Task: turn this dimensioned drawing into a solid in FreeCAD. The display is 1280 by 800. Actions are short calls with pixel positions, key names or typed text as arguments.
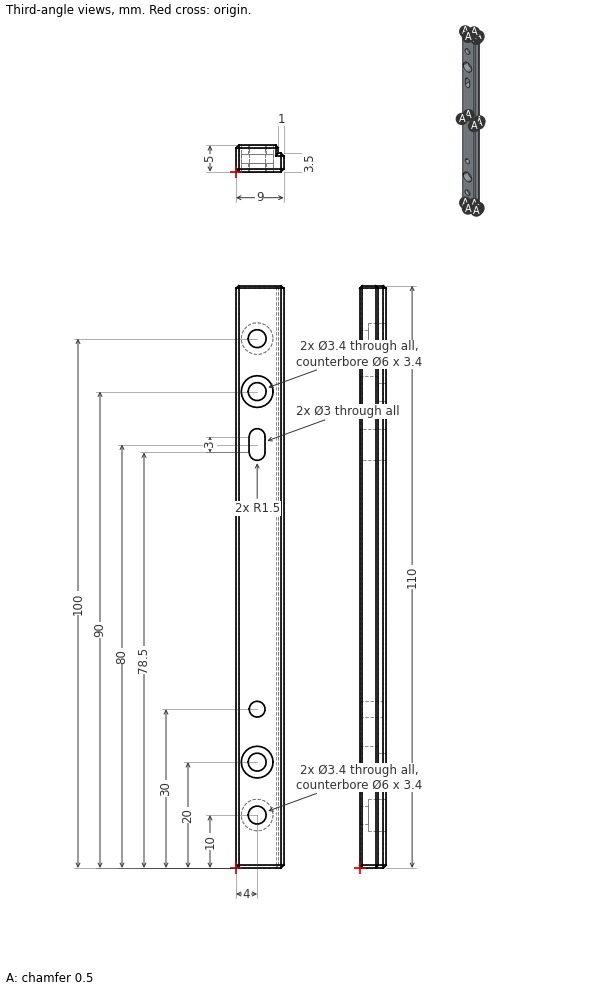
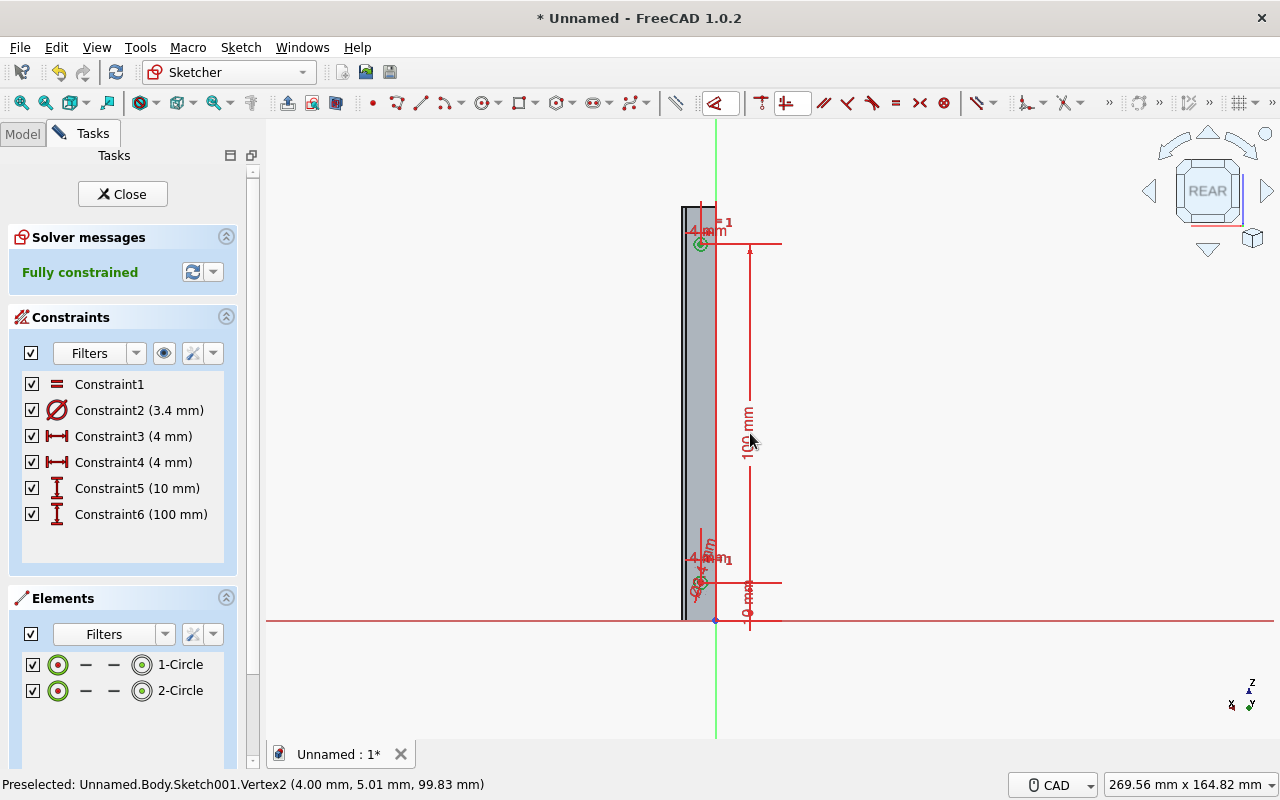
click(123, 194)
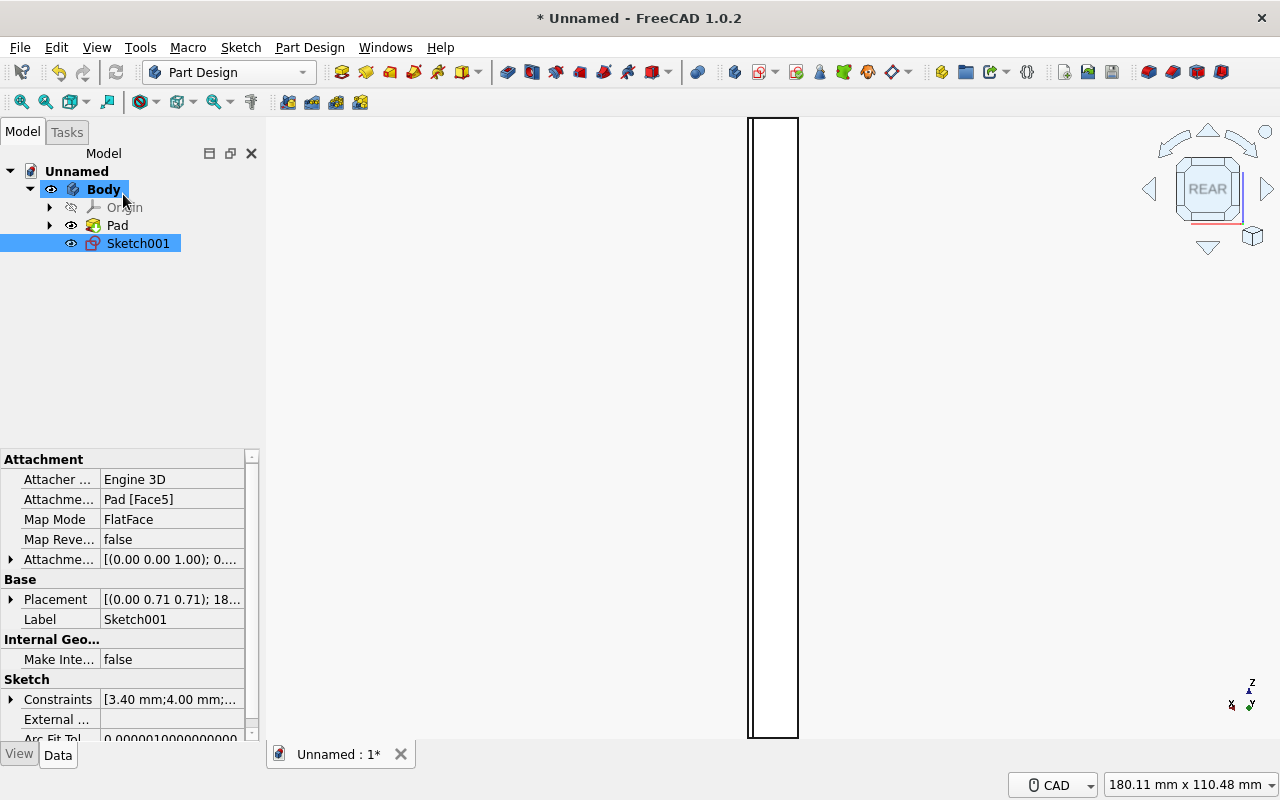
click(532, 72)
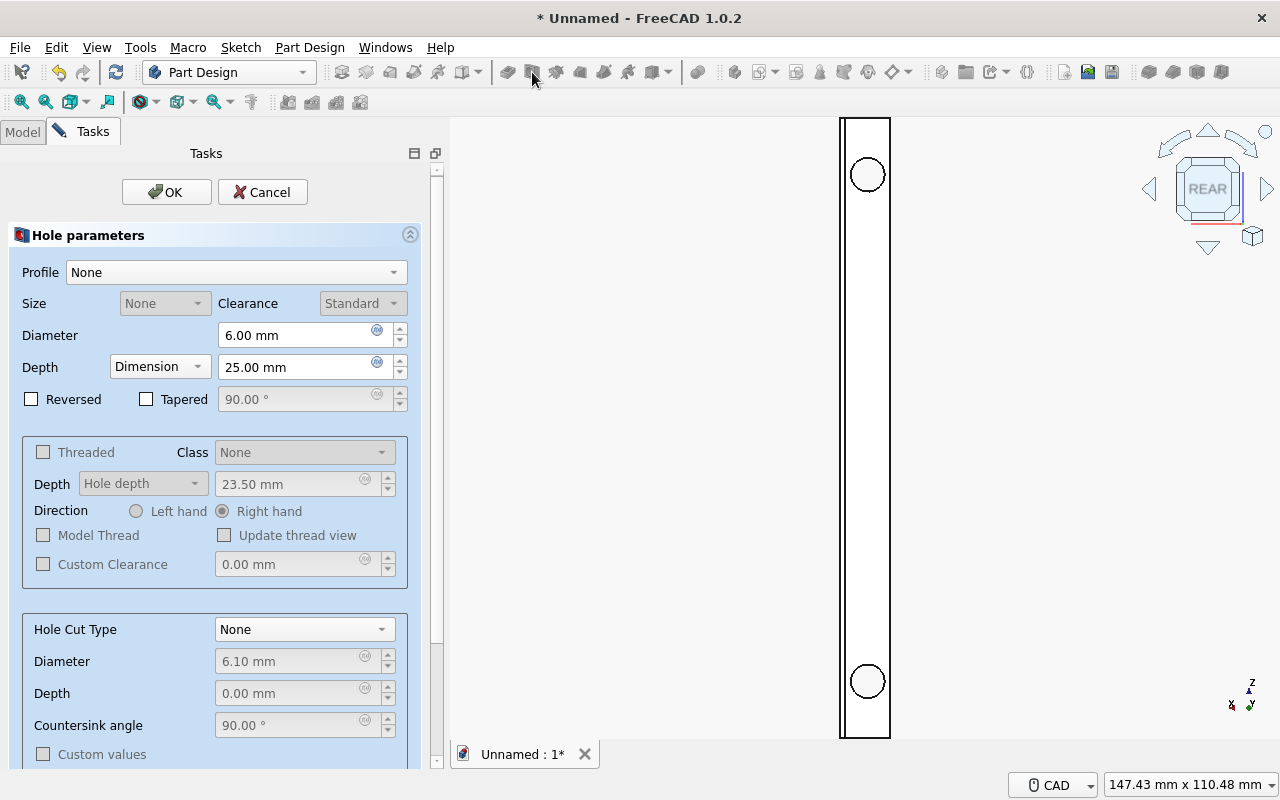
triple_click(305, 335)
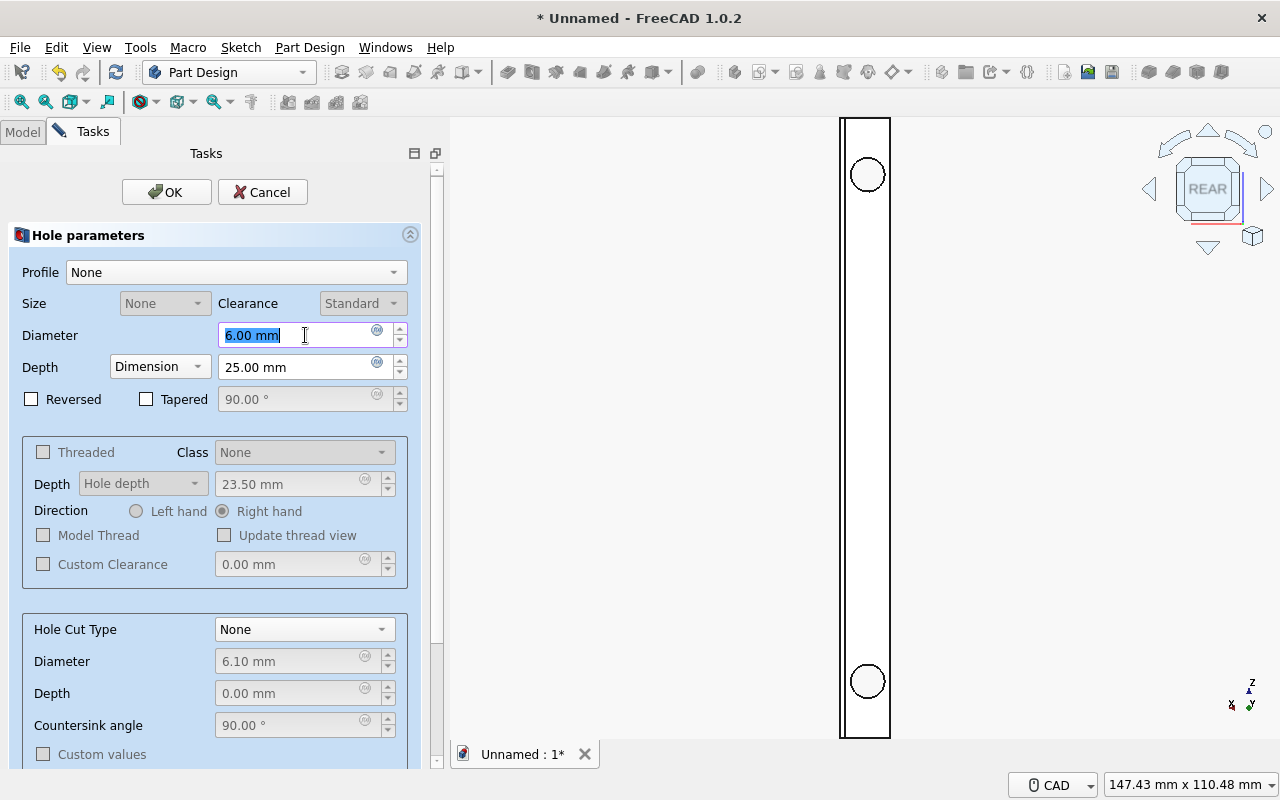
text(3.4)
key(Tab)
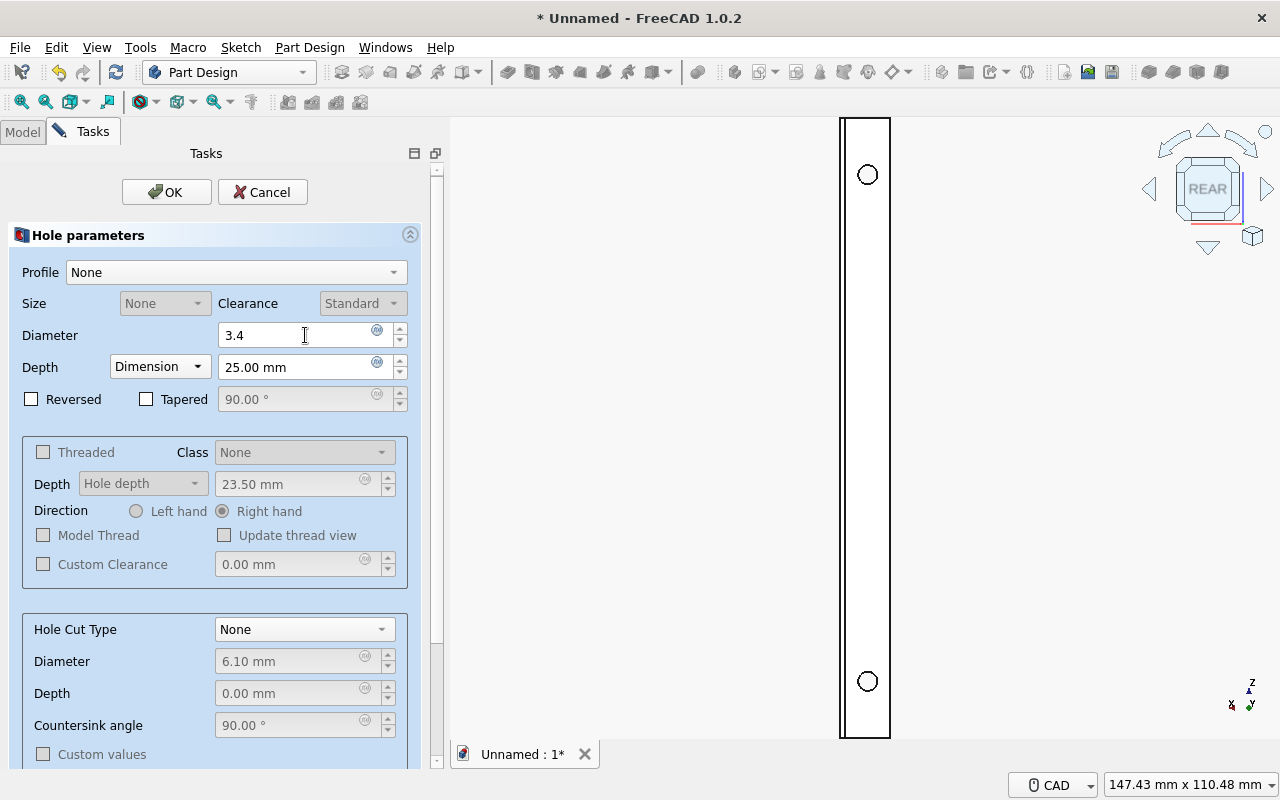
click(161, 366)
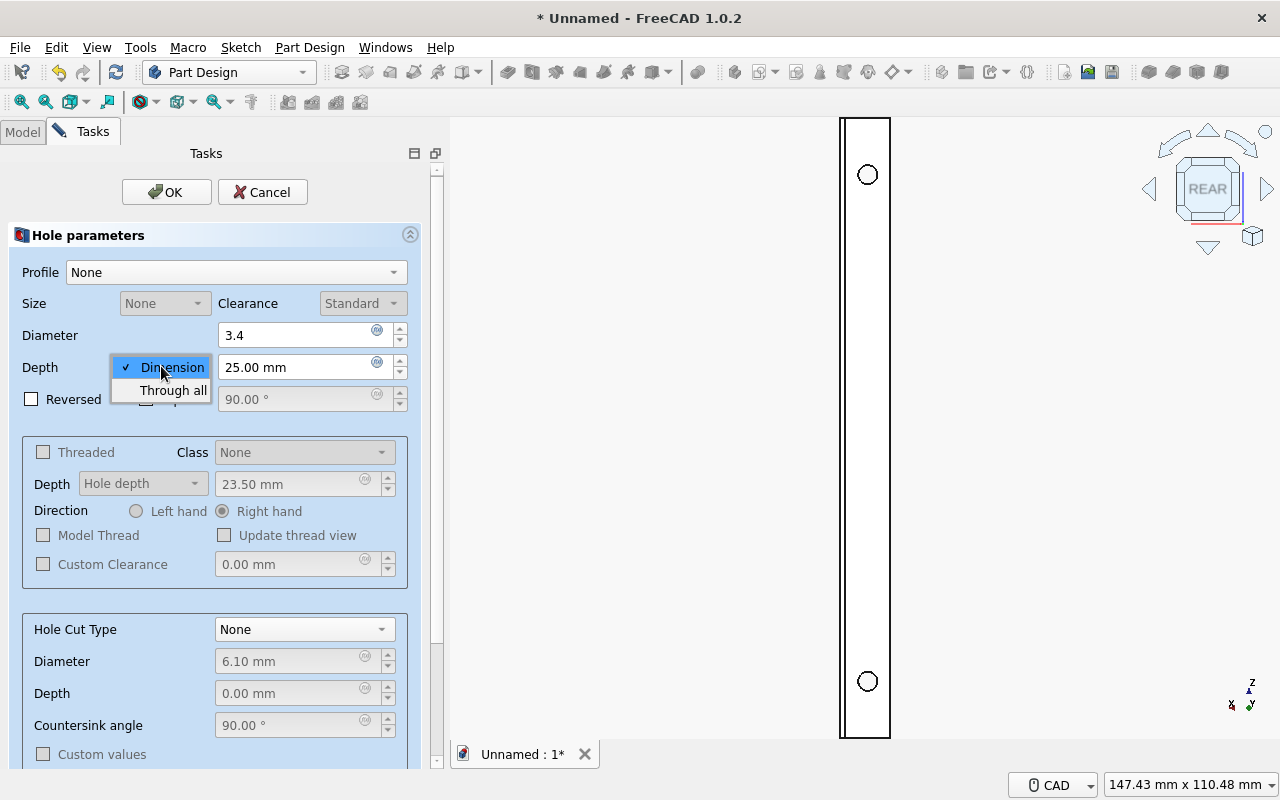
click(160, 390)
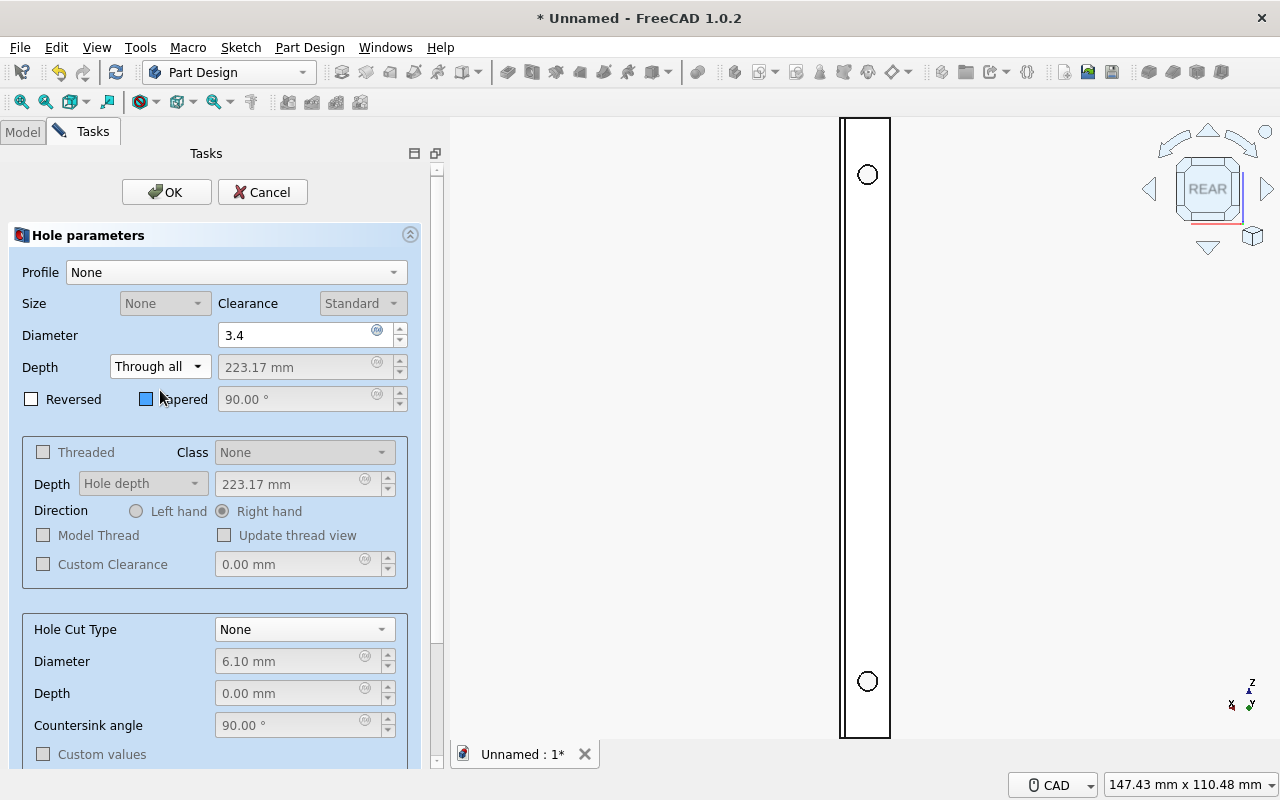
click(306, 630)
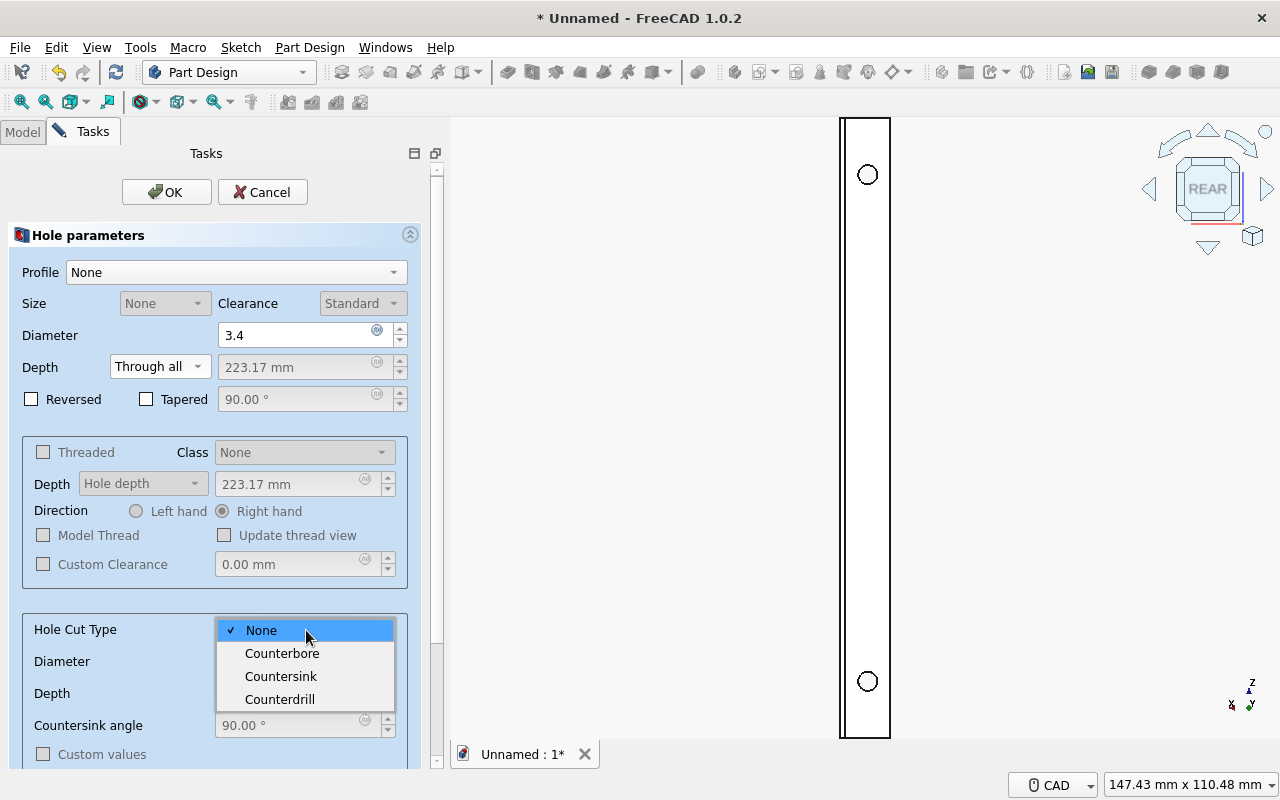
click(304, 654)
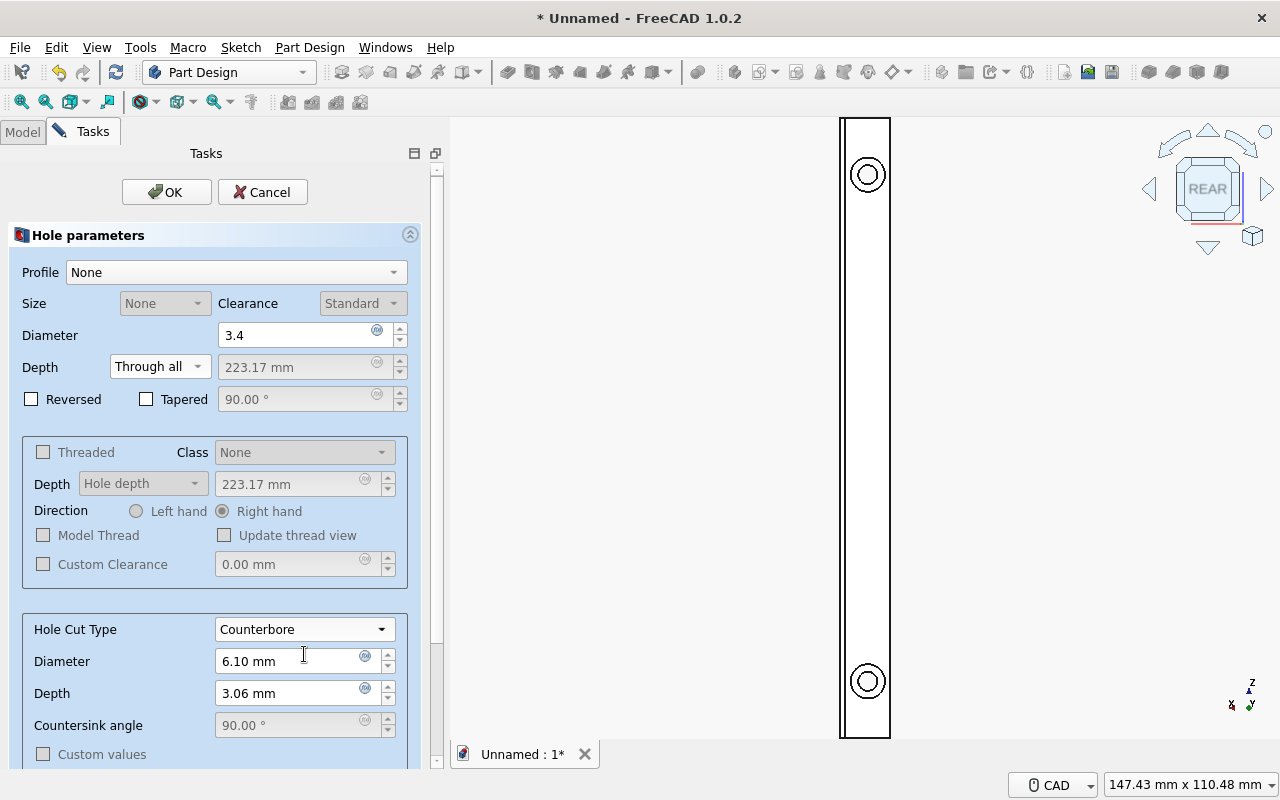
triple_click(298, 661)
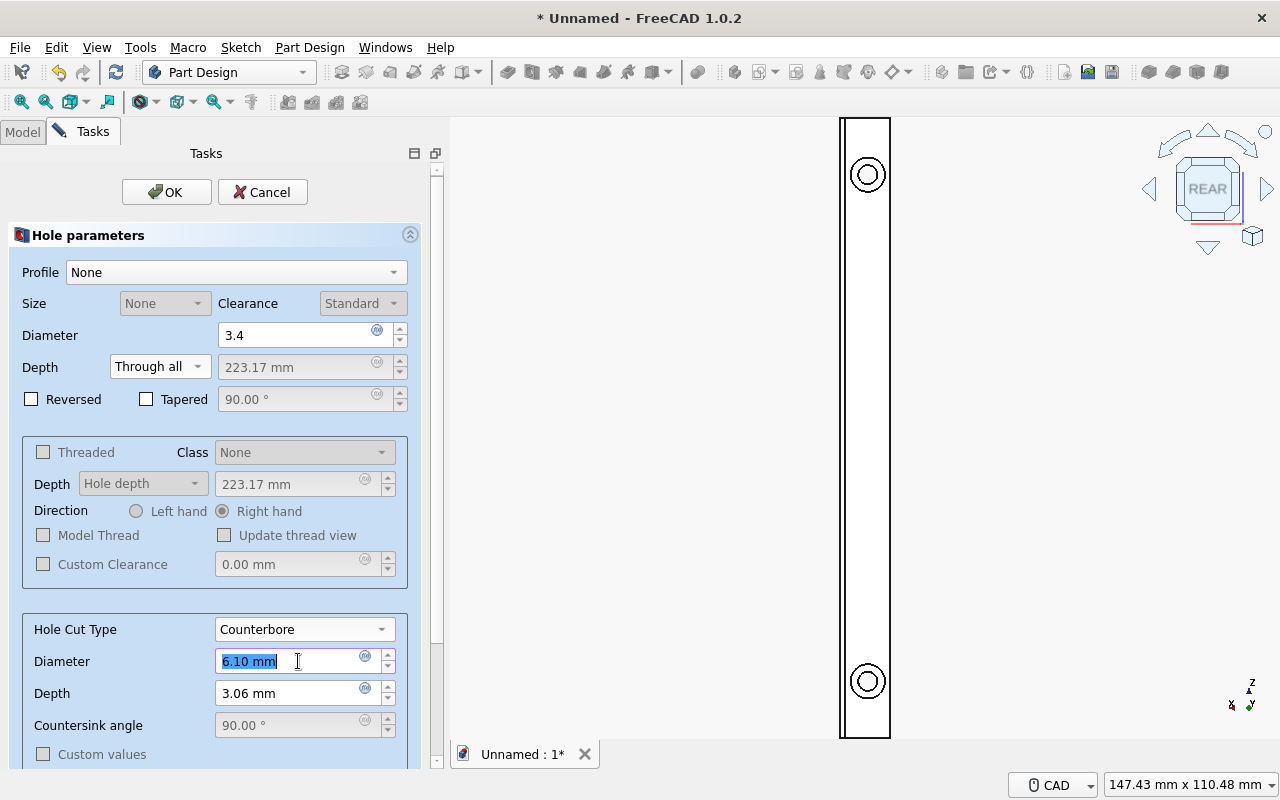
text(6)
key(Tab)